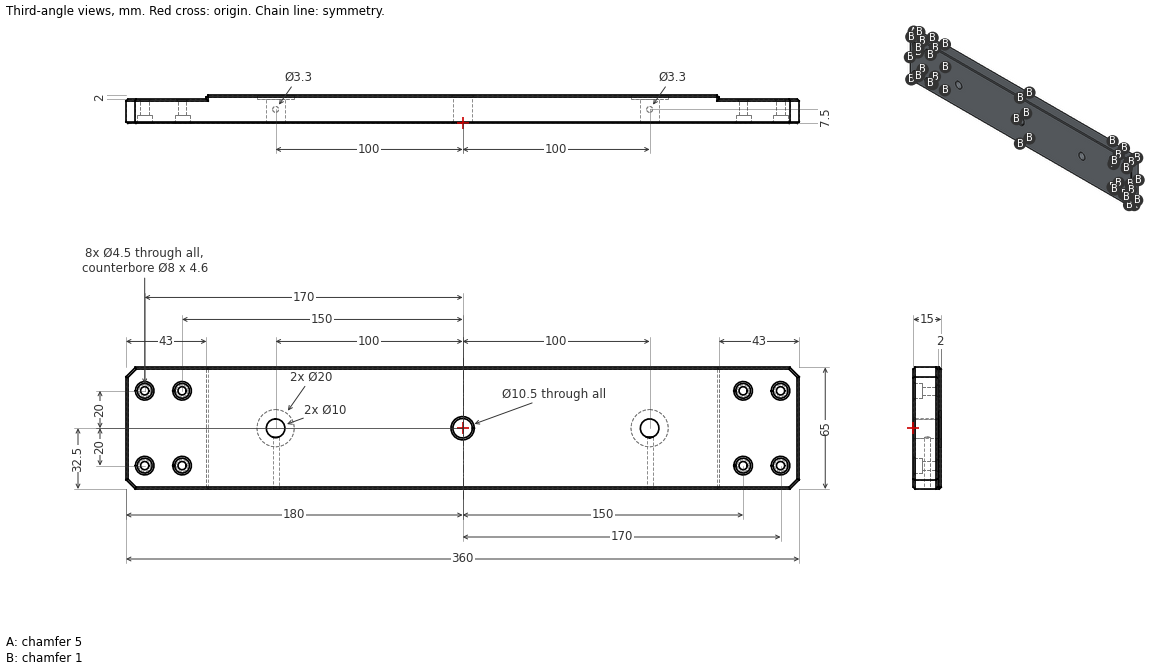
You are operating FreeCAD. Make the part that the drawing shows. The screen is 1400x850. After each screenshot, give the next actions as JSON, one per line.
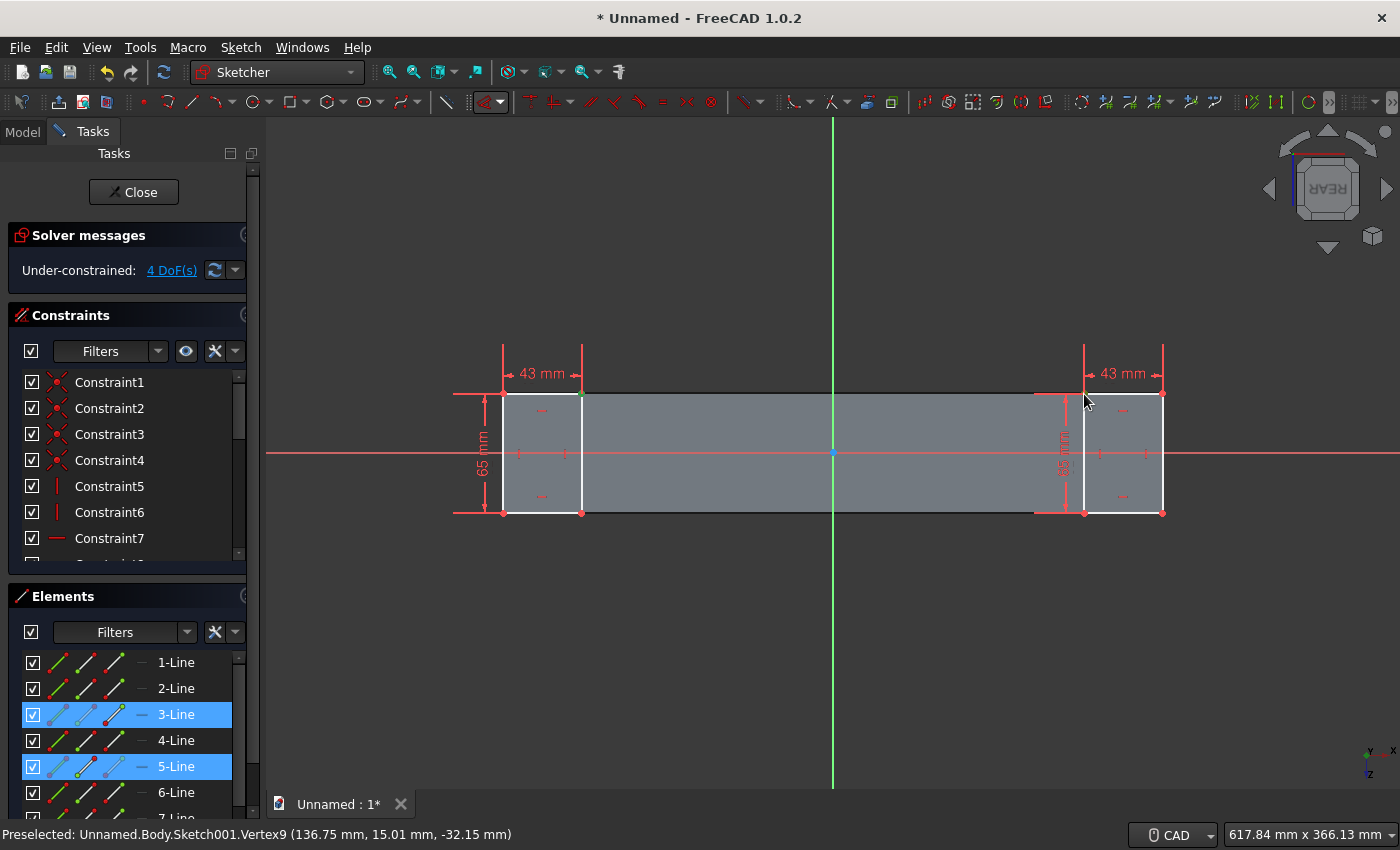
{"action": "left_click", "coordinate": [833, 717]}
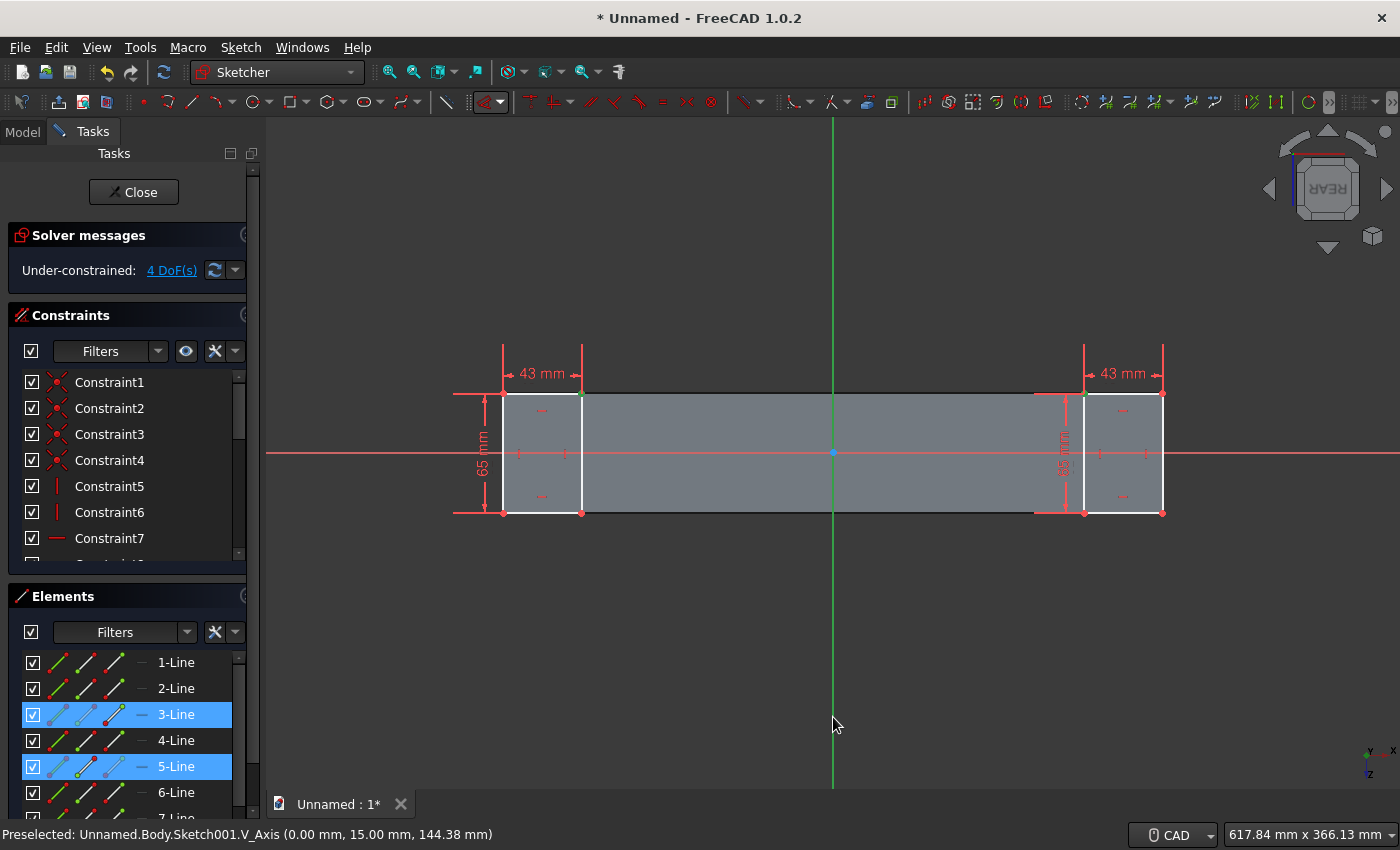
{"action": "left_click", "coordinate": [688, 102]}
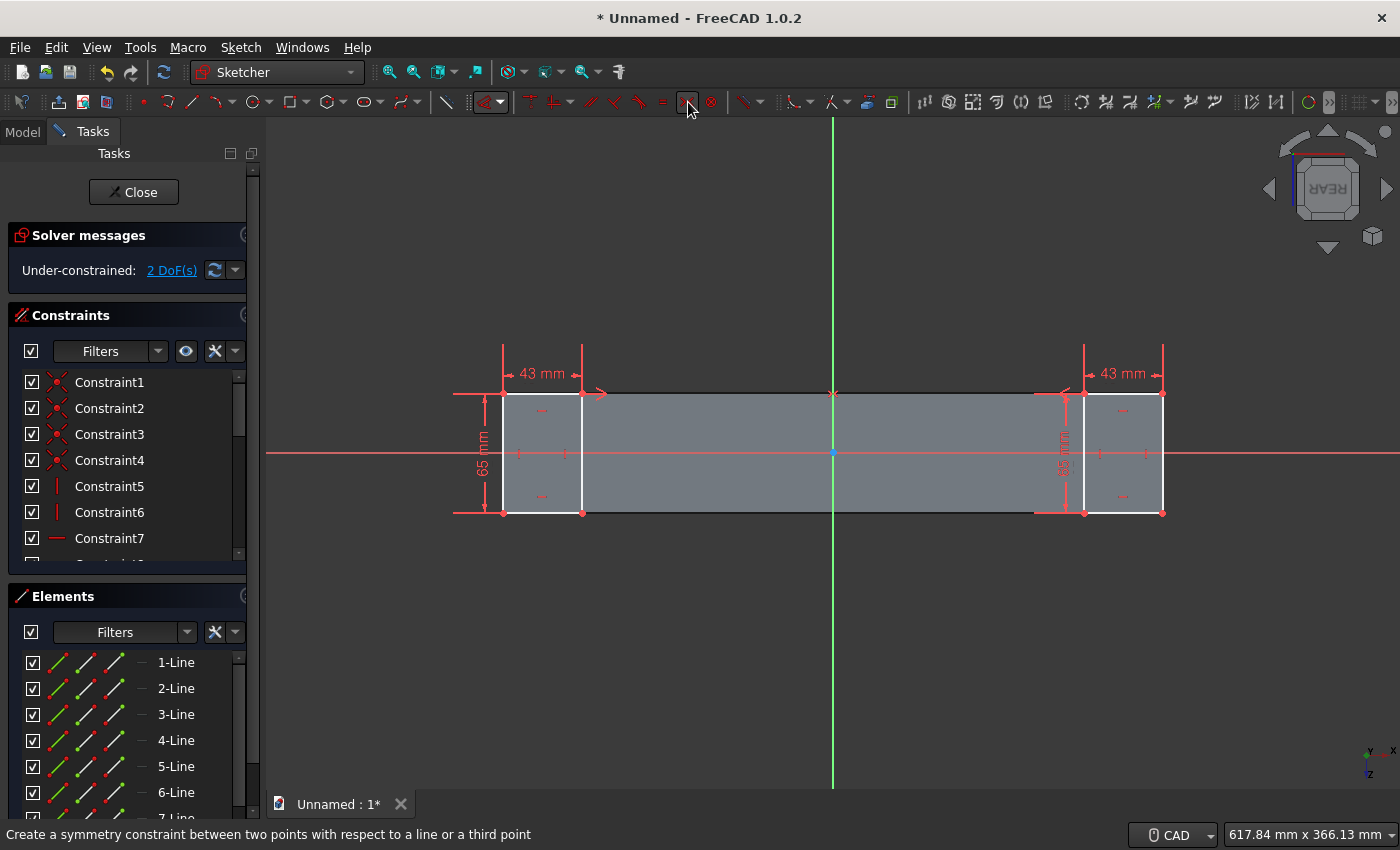
{"action": "left_click", "coordinate": [484, 102]}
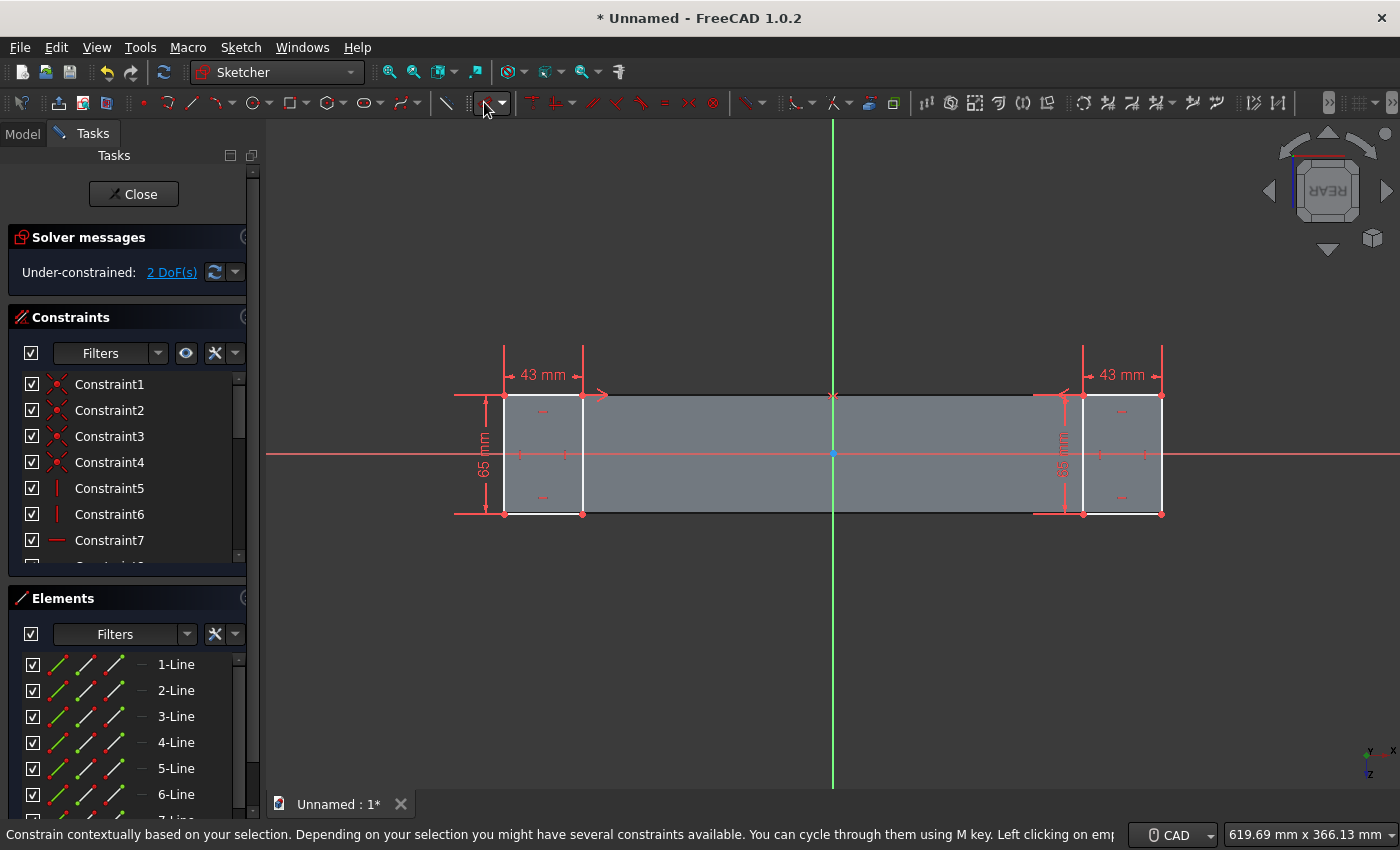
{"action": "left_click", "coordinate": [504, 395]}
{"action": "left_click", "coordinate": [669, 361]}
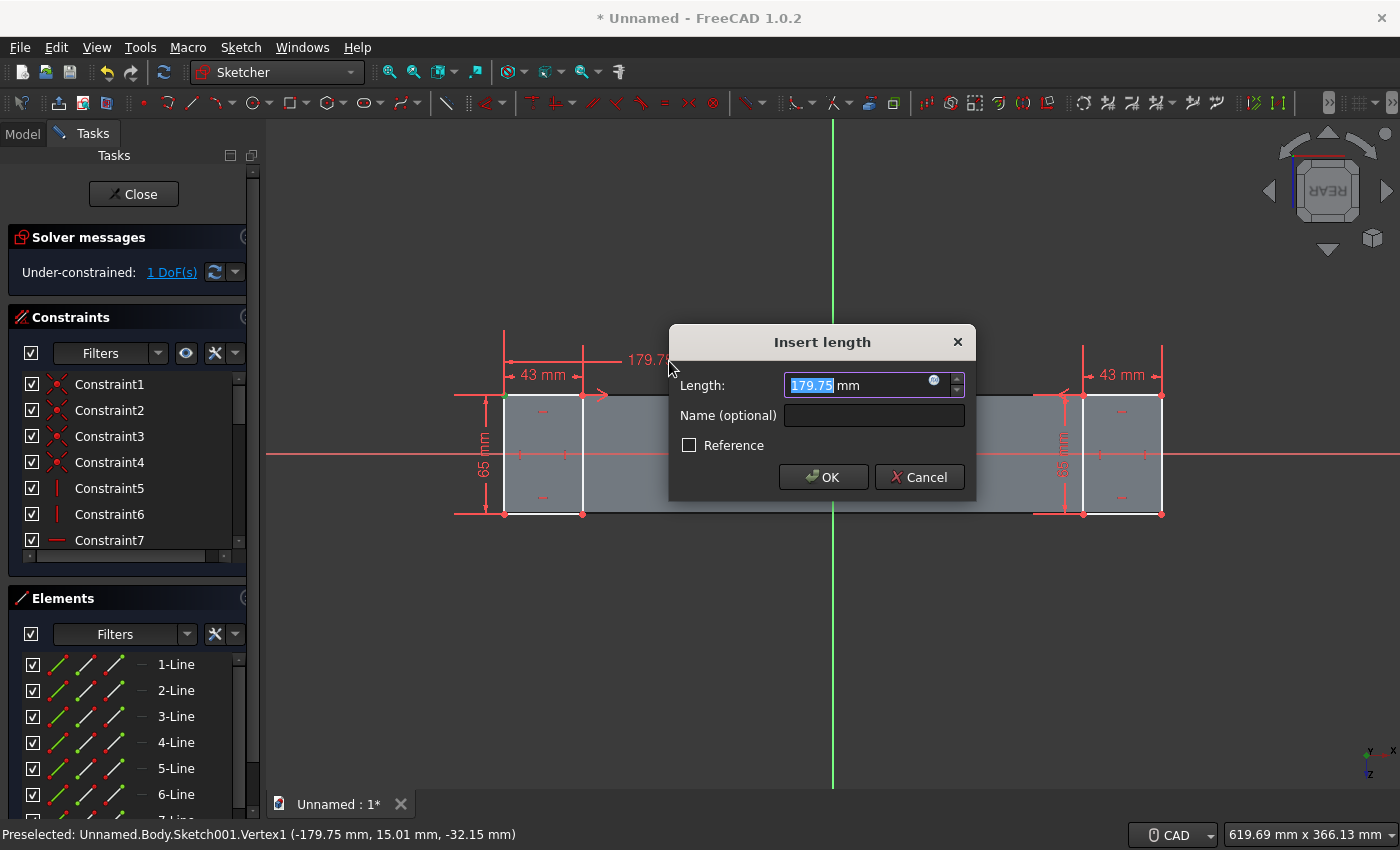
{"action": "type", "text": "180"}
{"action": "key", "text": "Return"}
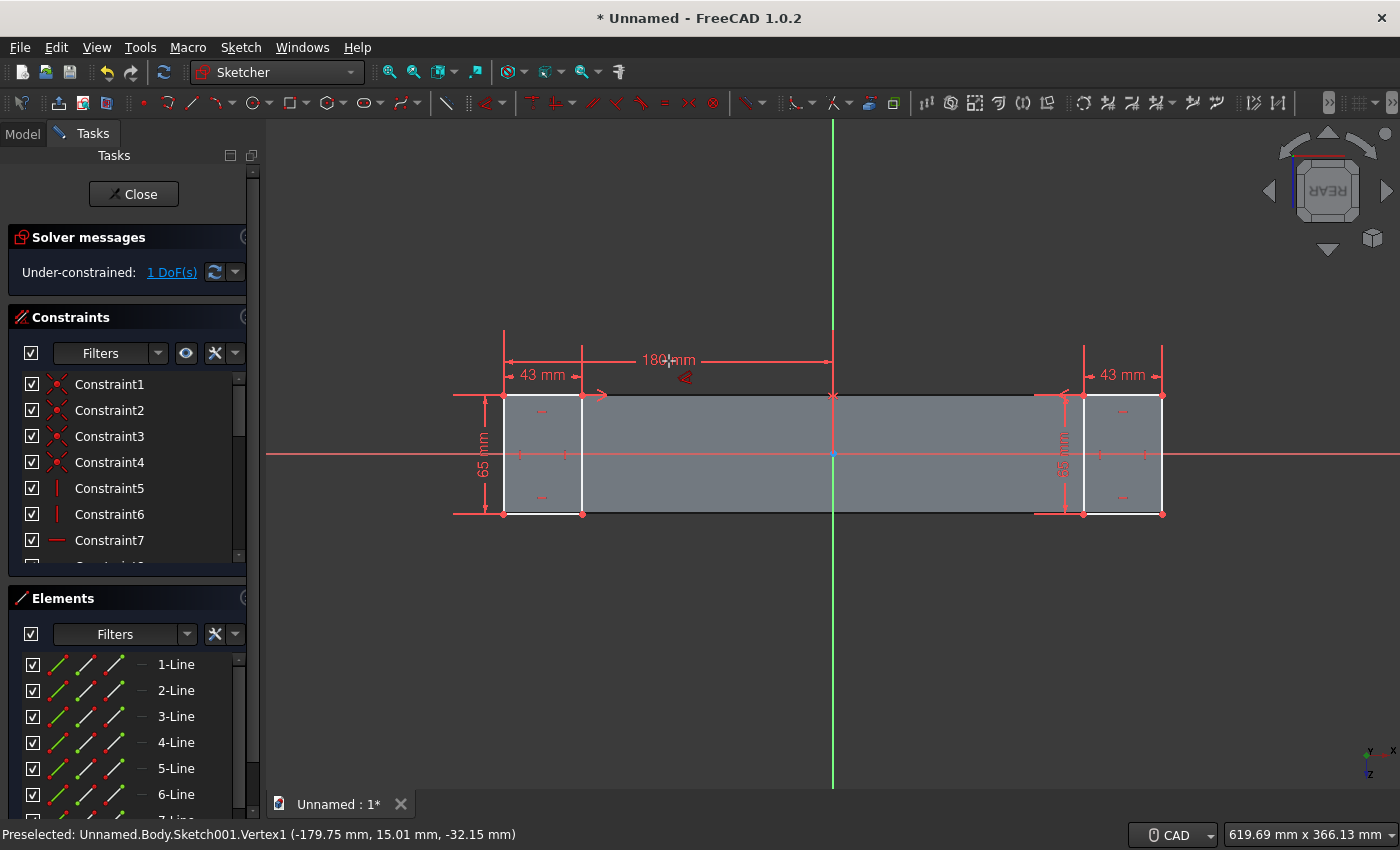
{"action": "left_click", "coordinate": [504, 395]}
{"action": "left_click", "coordinate": [470, 425]}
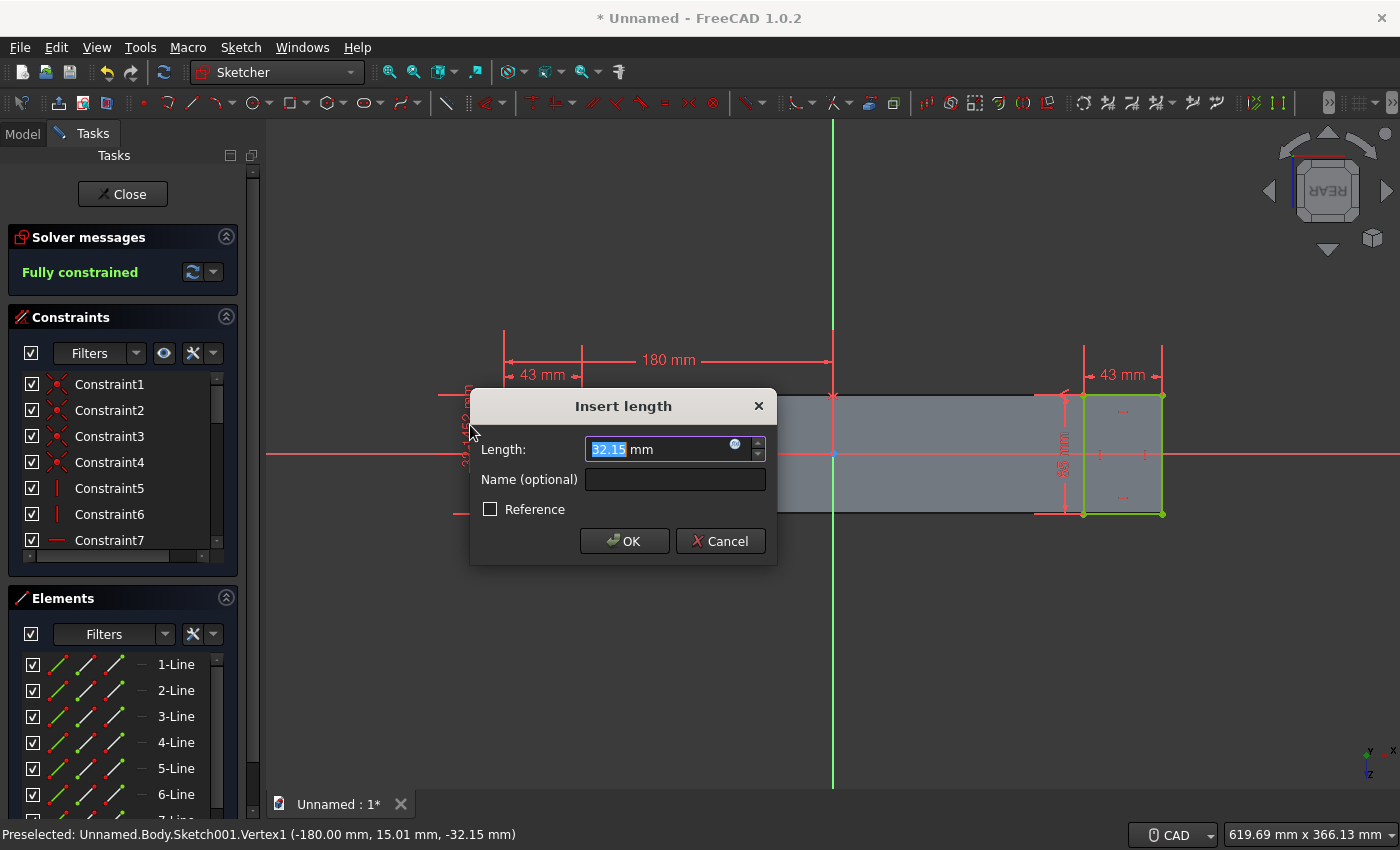
{"action": "type", "text": "32.5"}
{"action": "key", "text": "Return"}
{"action": "key", "text": "Escape"}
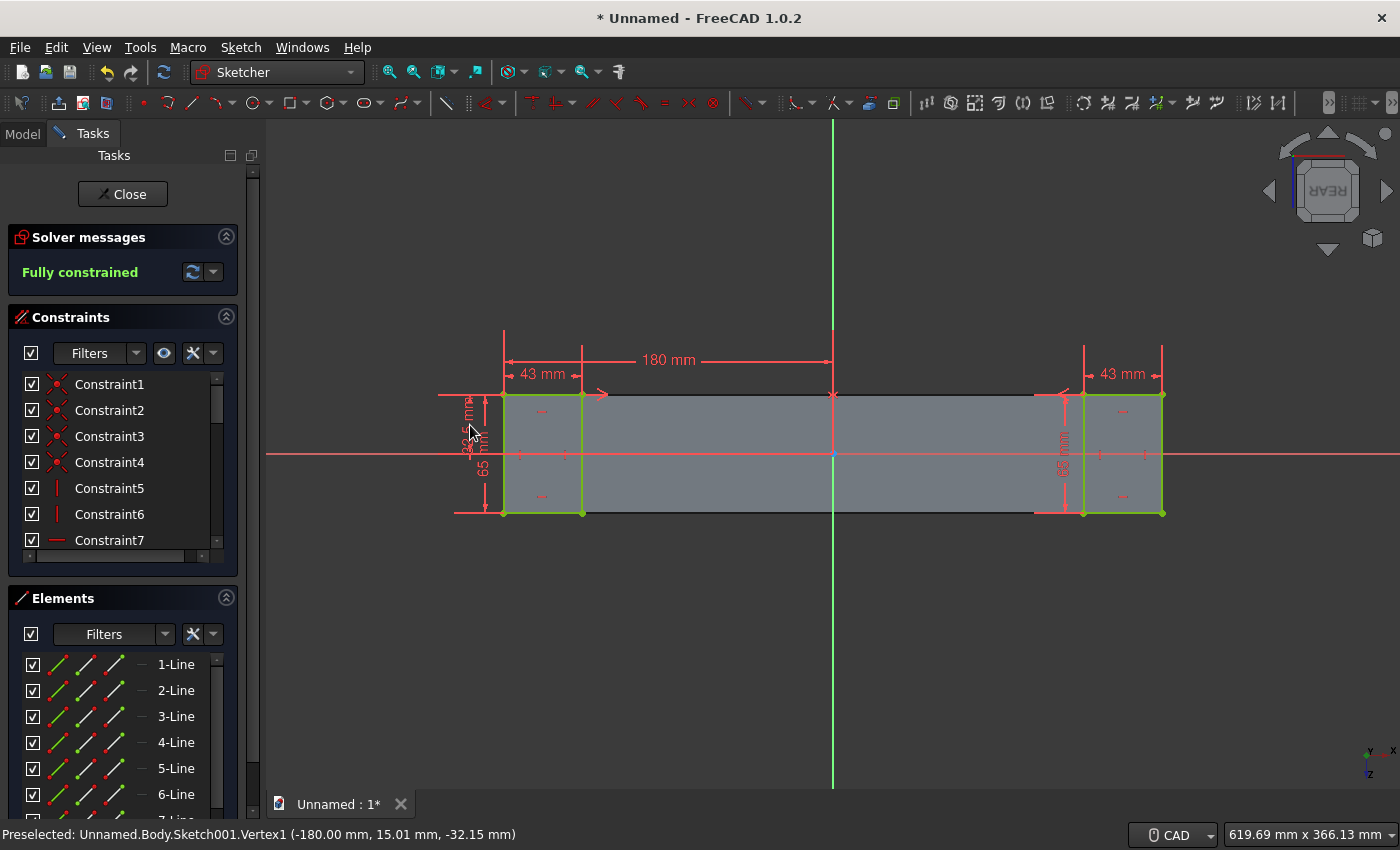
{"action": "left_click", "coordinate": [123, 194]}